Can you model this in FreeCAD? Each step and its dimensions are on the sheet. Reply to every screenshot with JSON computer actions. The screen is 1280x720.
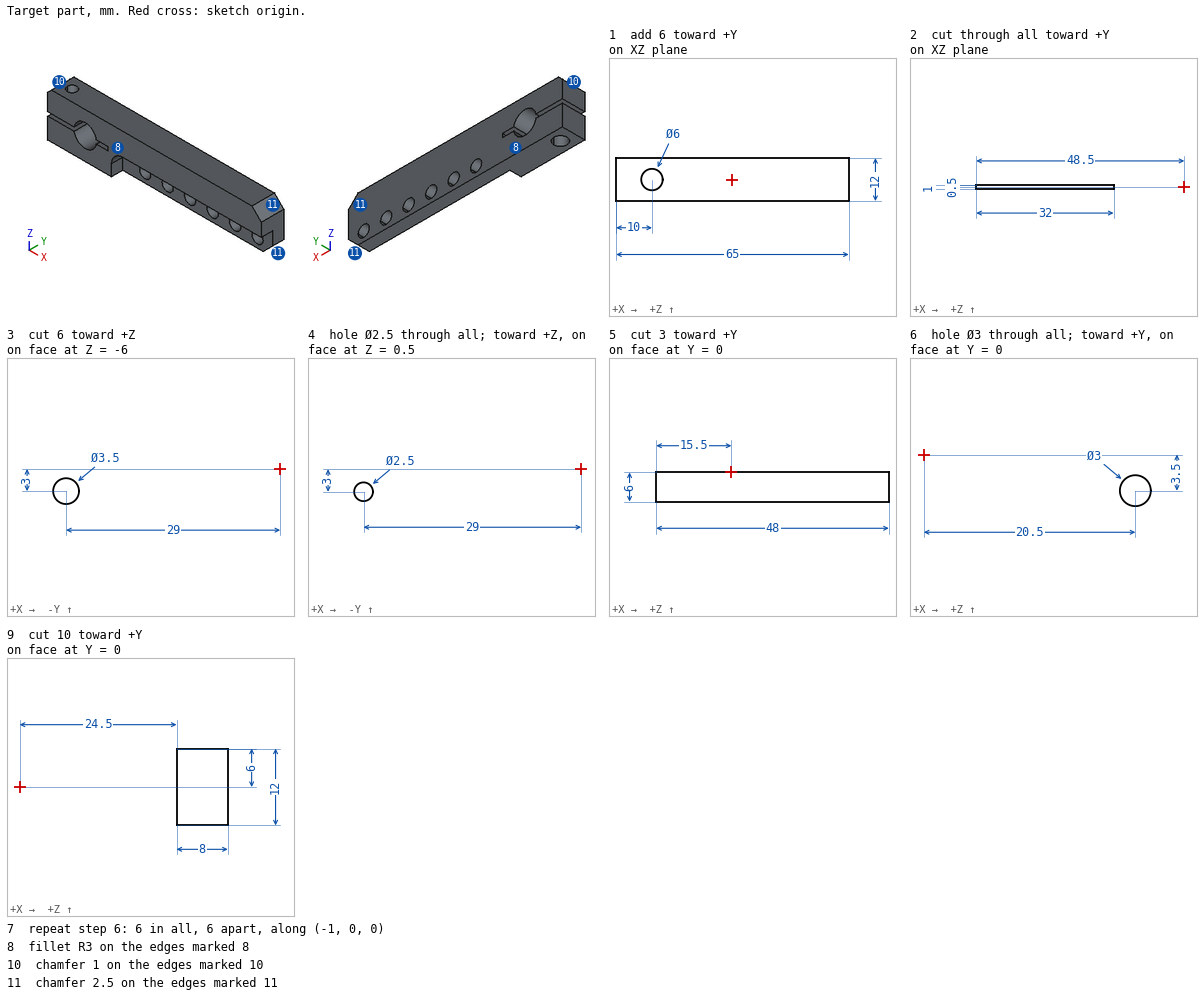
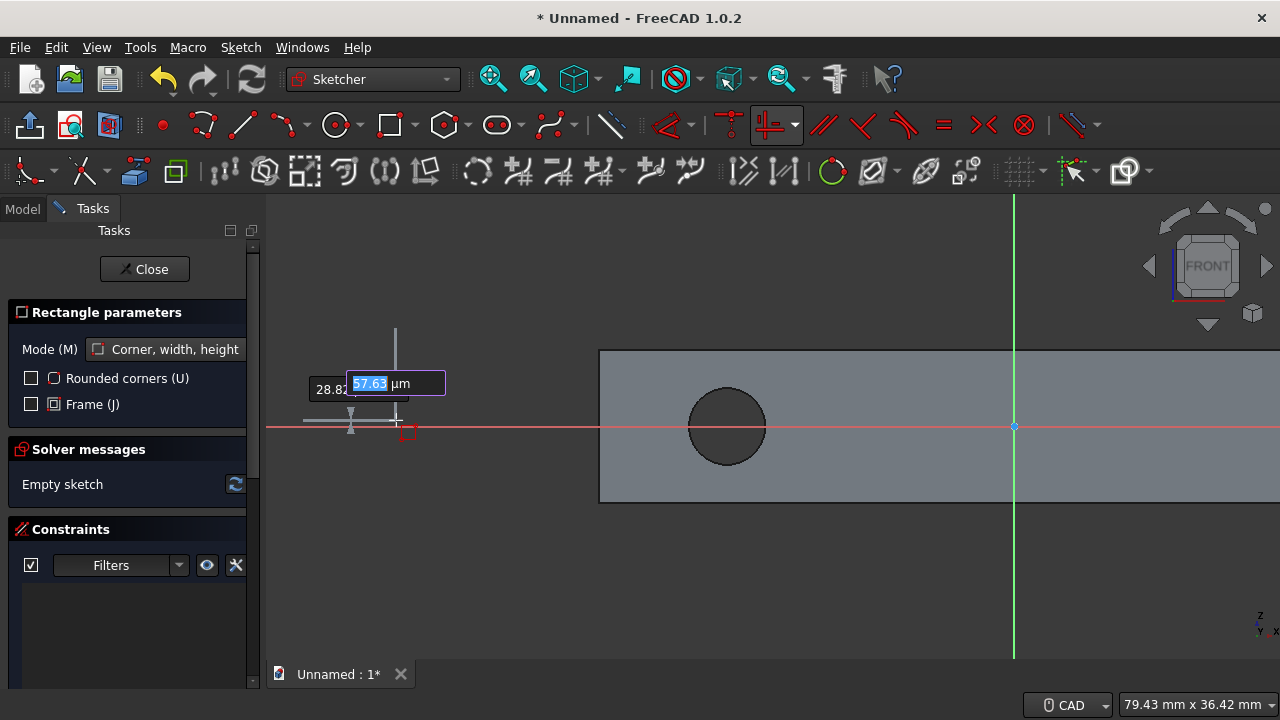
{"action": "scroll", "coordinate": [804, 433], "scroll_direction": "up", "scroll_amount": 5}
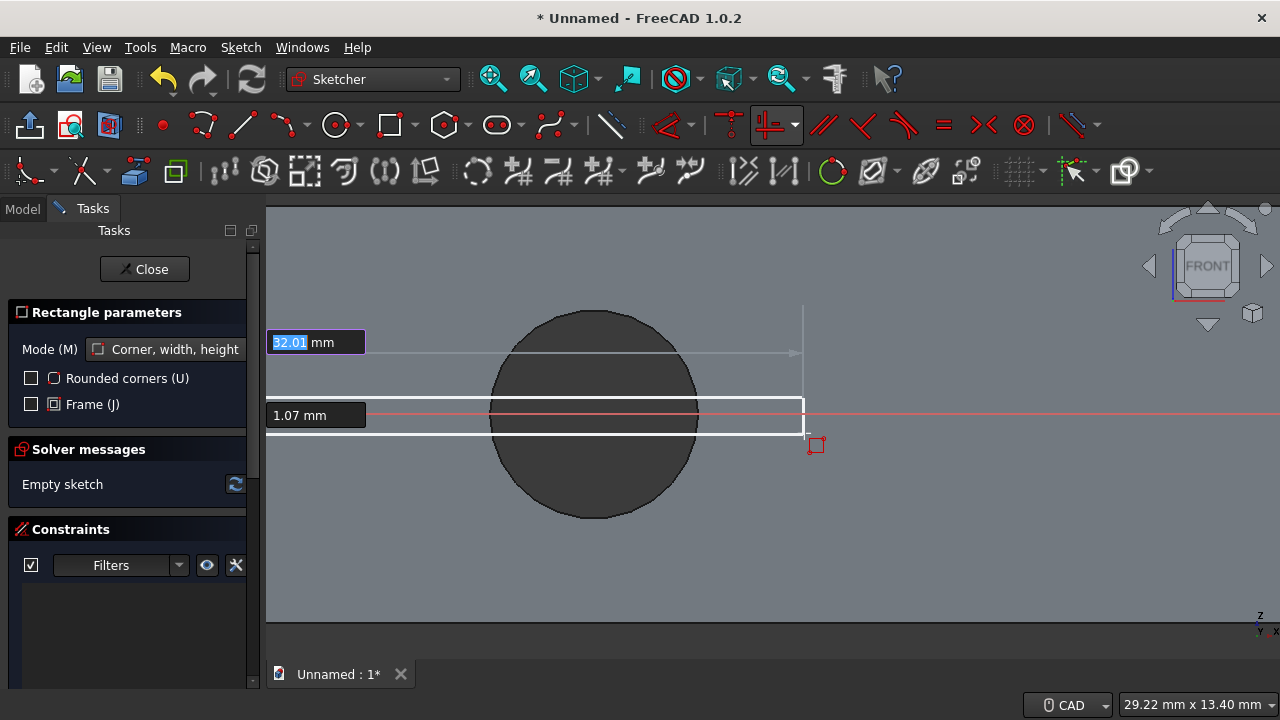
{"action": "left_click", "coordinate": [802, 432]}
{"action": "key", "text": "Escape"}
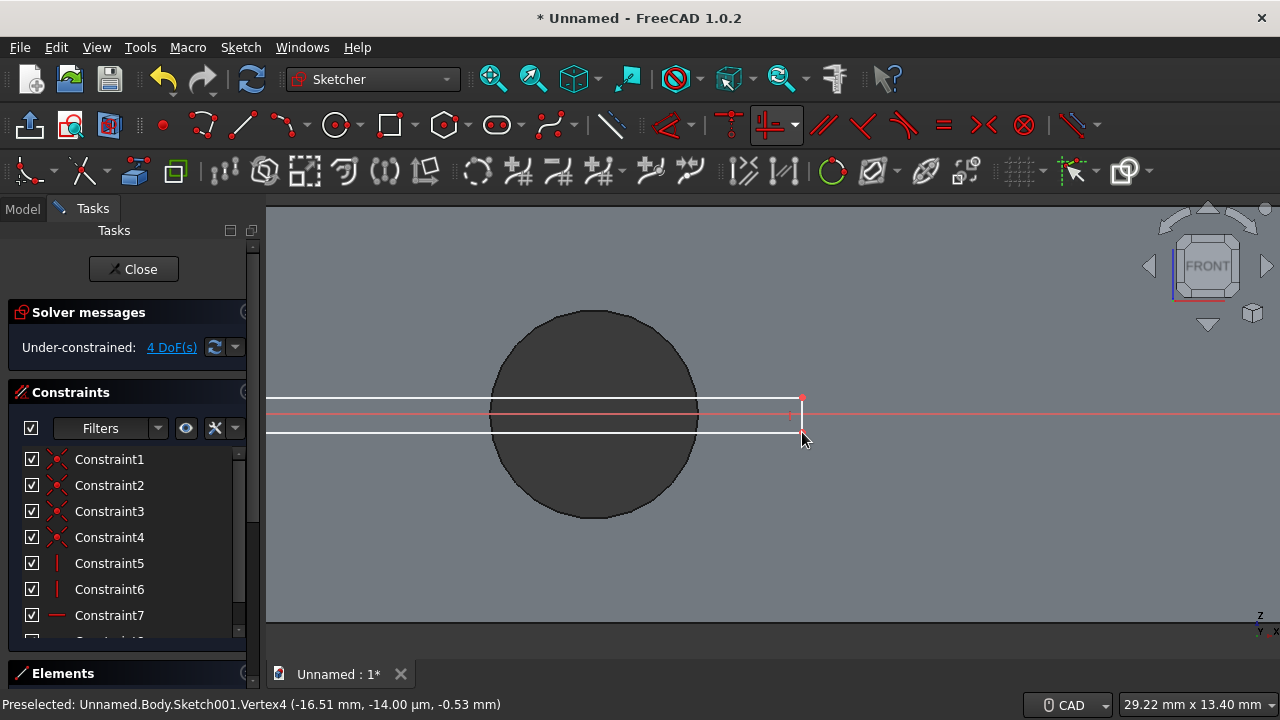
{"action": "left_click", "coordinate": [666, 126]}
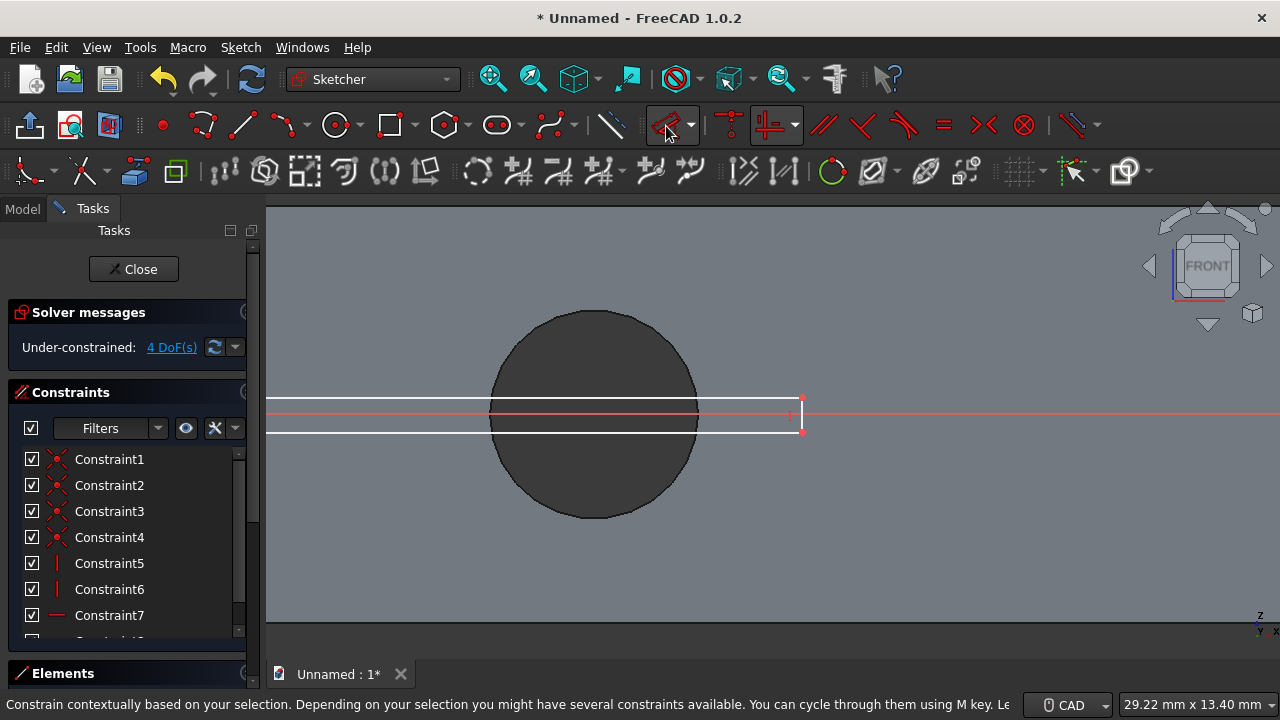
{"action": "scroll", "coordinate": [804, 434], "scroll_direction": "down", "scroll_amount": 5}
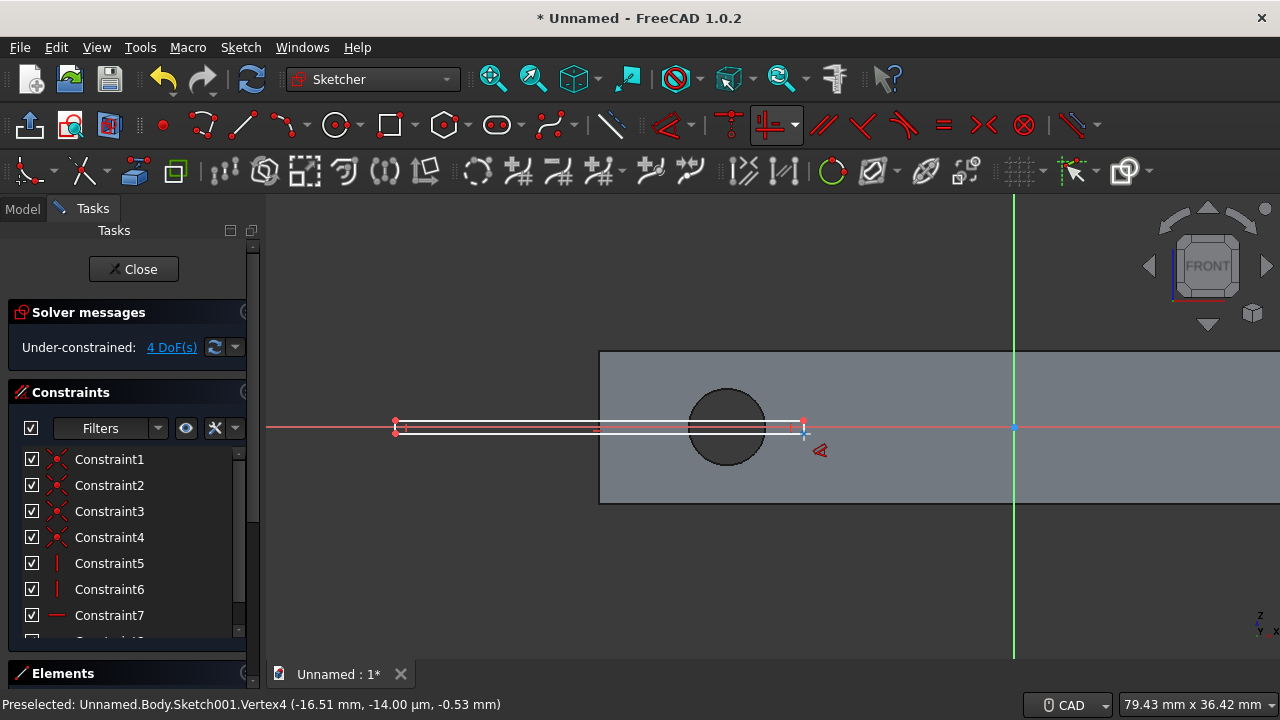
{"action": "scroll", "coordinate": [395, 426], "scroll_direction": "up", "scroll_amount": 6}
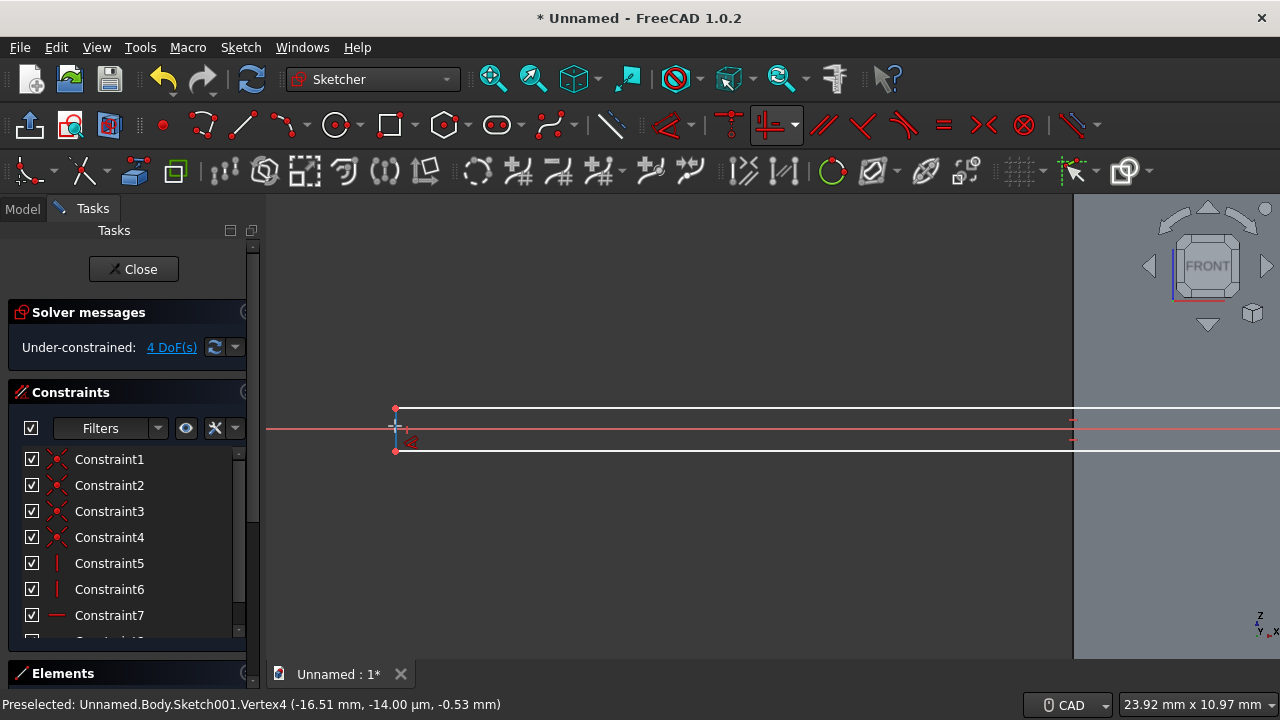
{"action": "left_click", "coordinate": [396, 425]}
{"action": "left_click", "coordinate": [362, 415]}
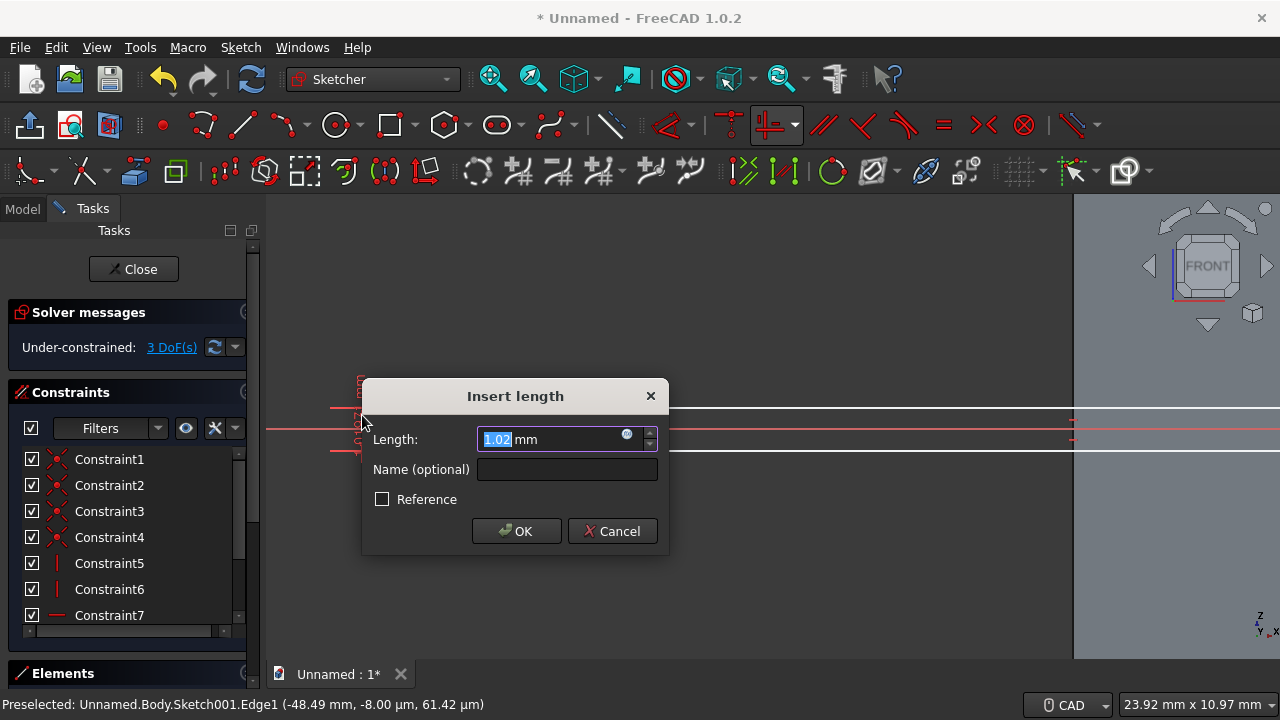
{"action": "type", "text": "1"}
{"action": "key", "text": "Return"}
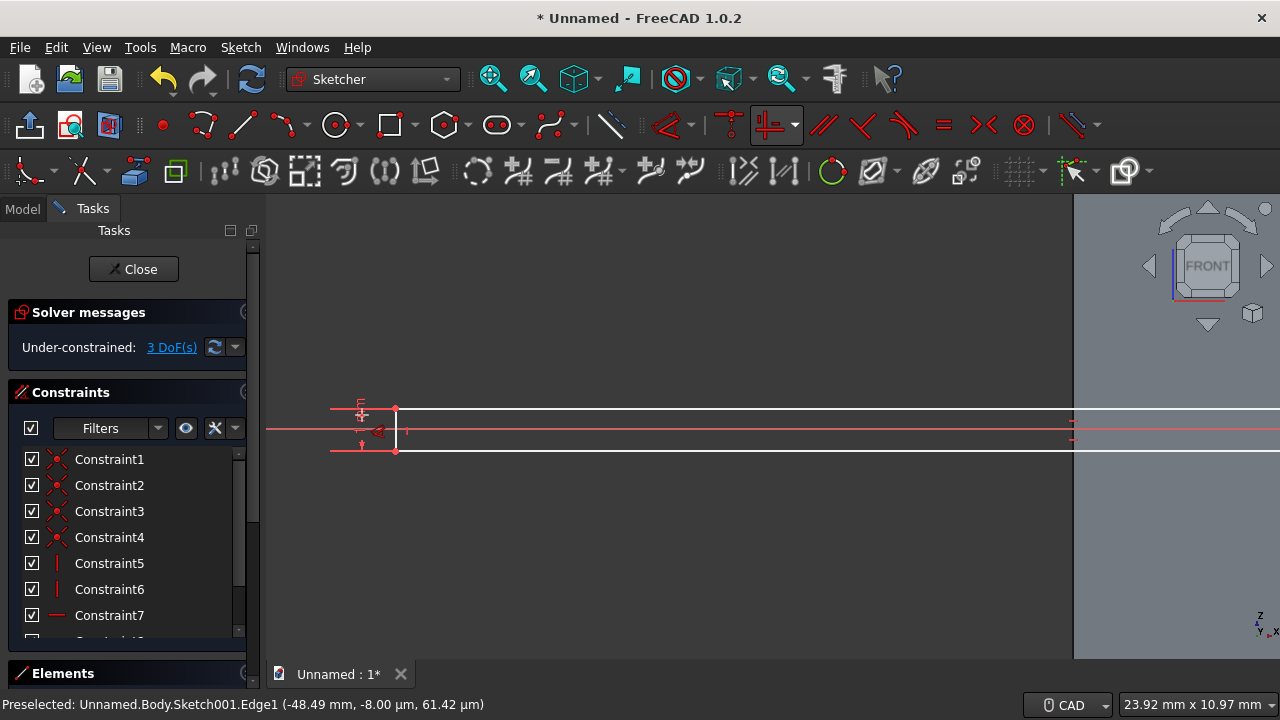
{"action": "left_click", "coordinate": [802, 451]}
{"action": "left_click", "coordinate": [755, 485]}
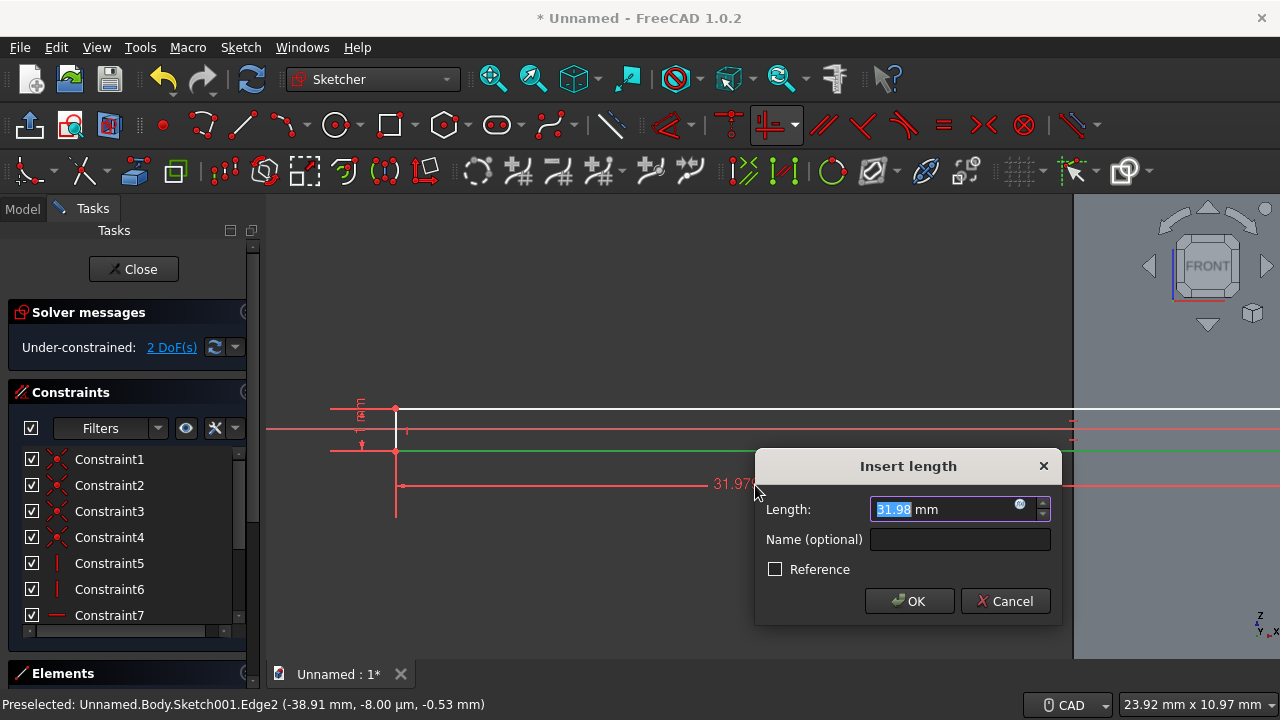
{"action": "type", "text": "32"}
{"action": "key", "text": "Return"}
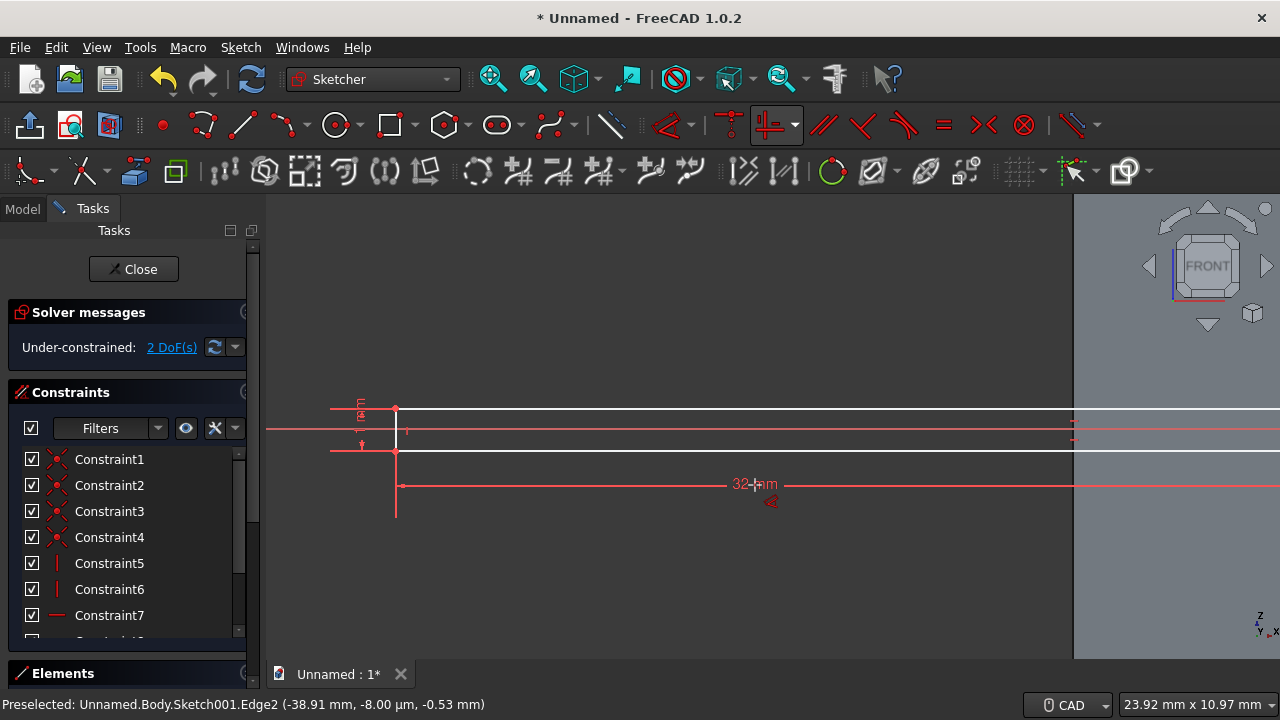
{"action": "scroll", "coordinate": [396, 409], "scroll_direction": "up", "scroll_amount": 4}